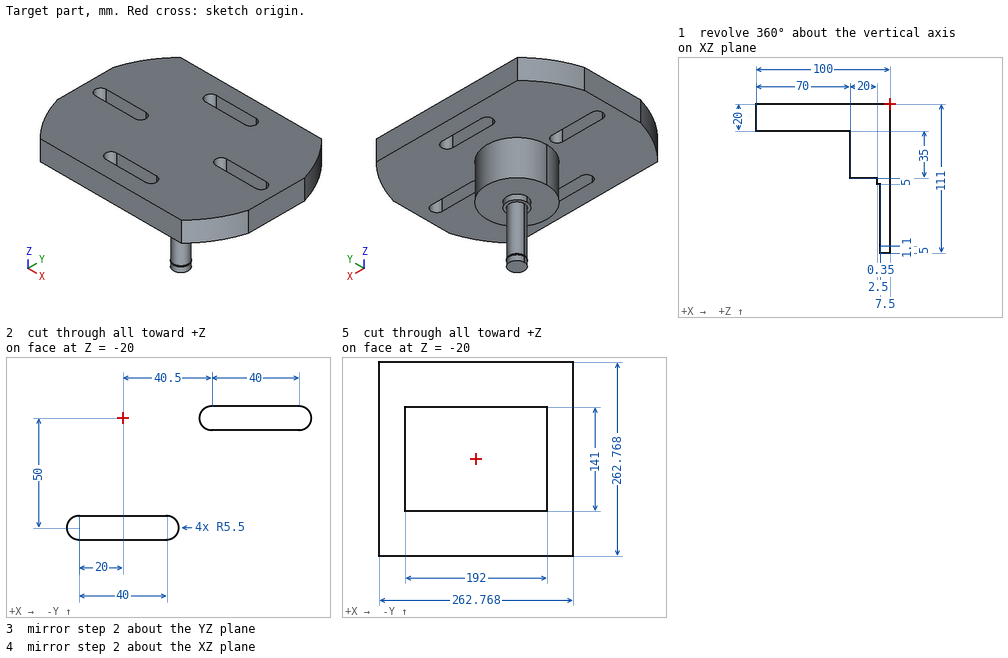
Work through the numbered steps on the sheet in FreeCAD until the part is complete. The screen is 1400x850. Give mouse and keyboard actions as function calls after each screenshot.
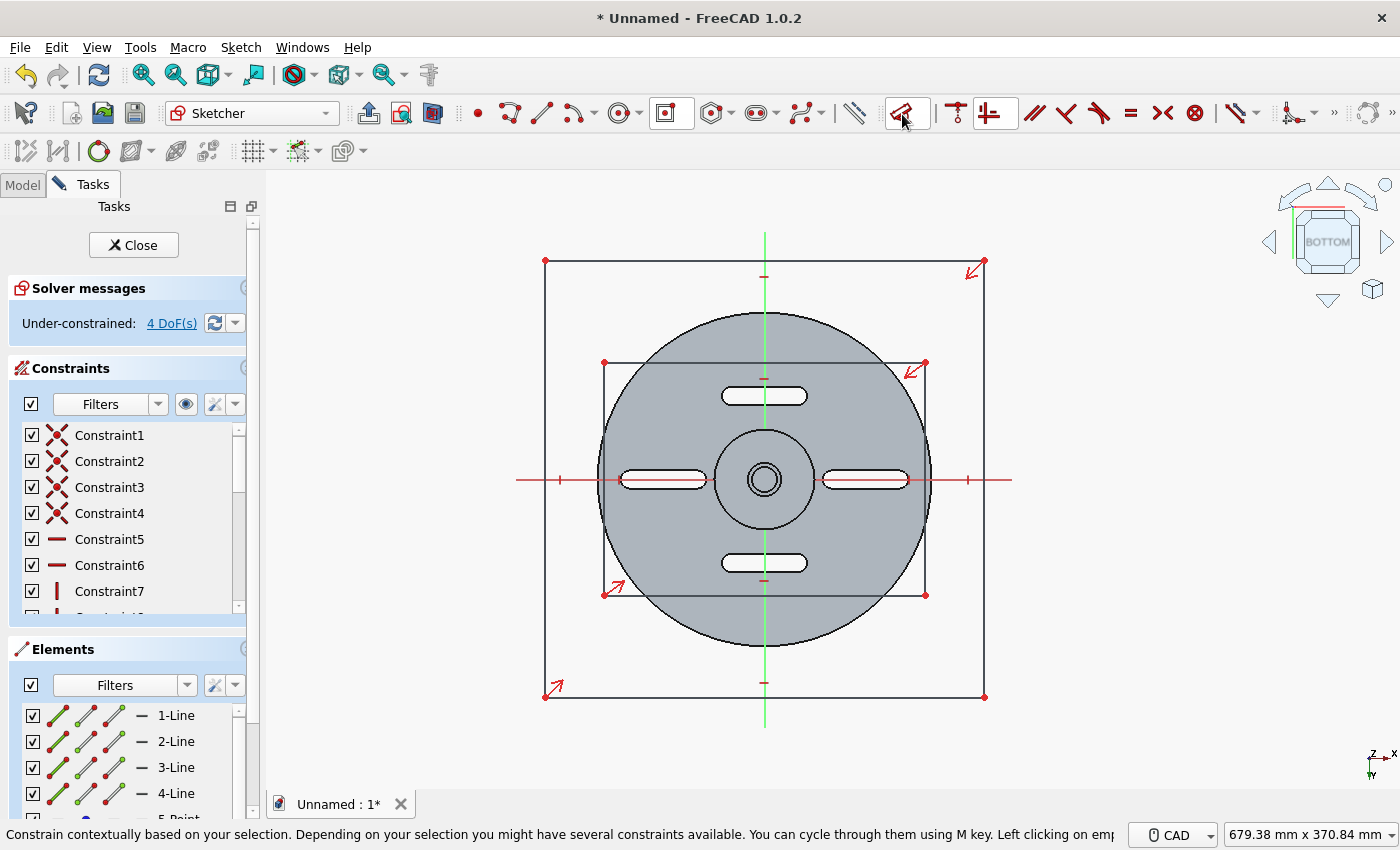
click(700, 596)
click(691, 630)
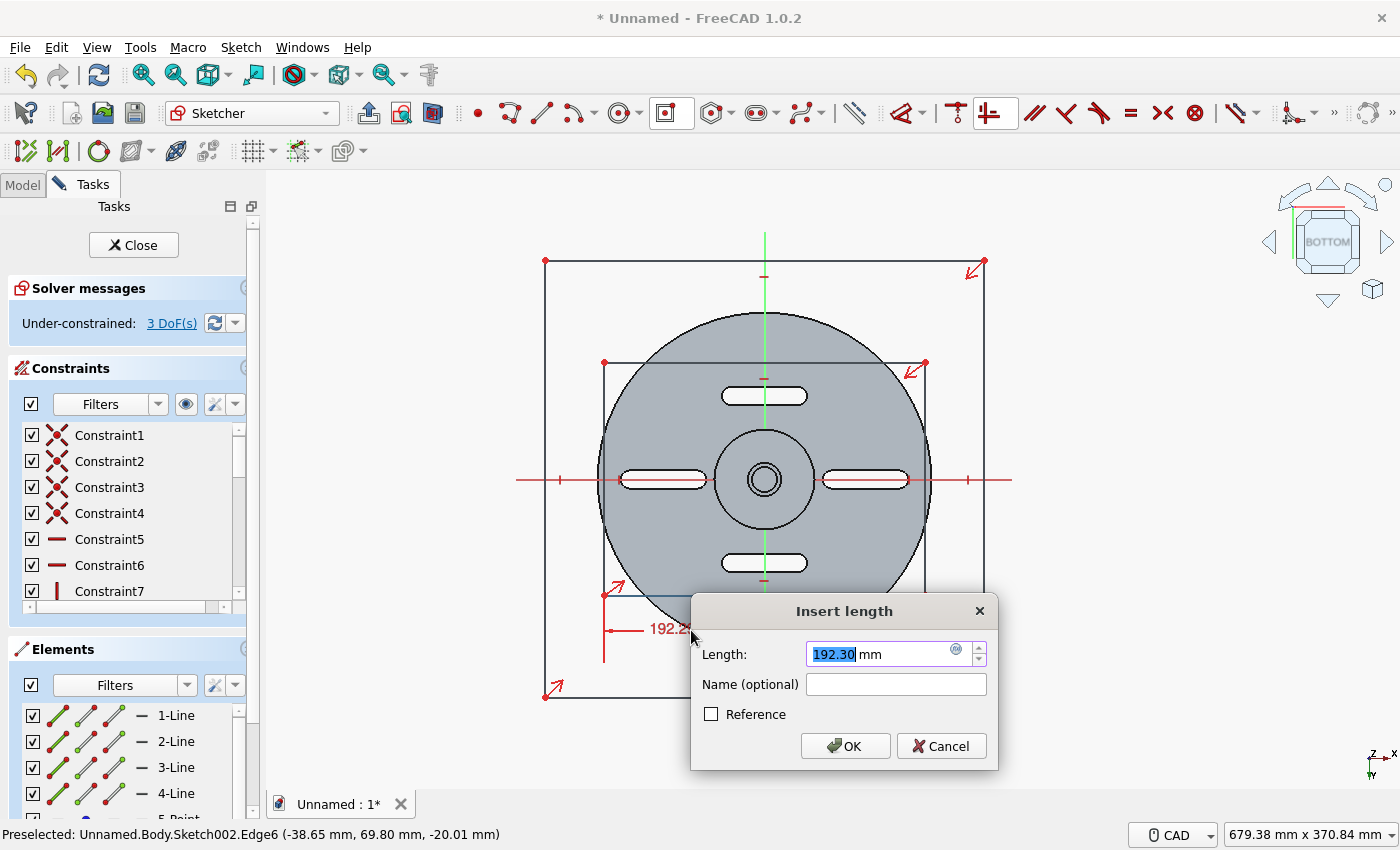
text(192)
key(Return)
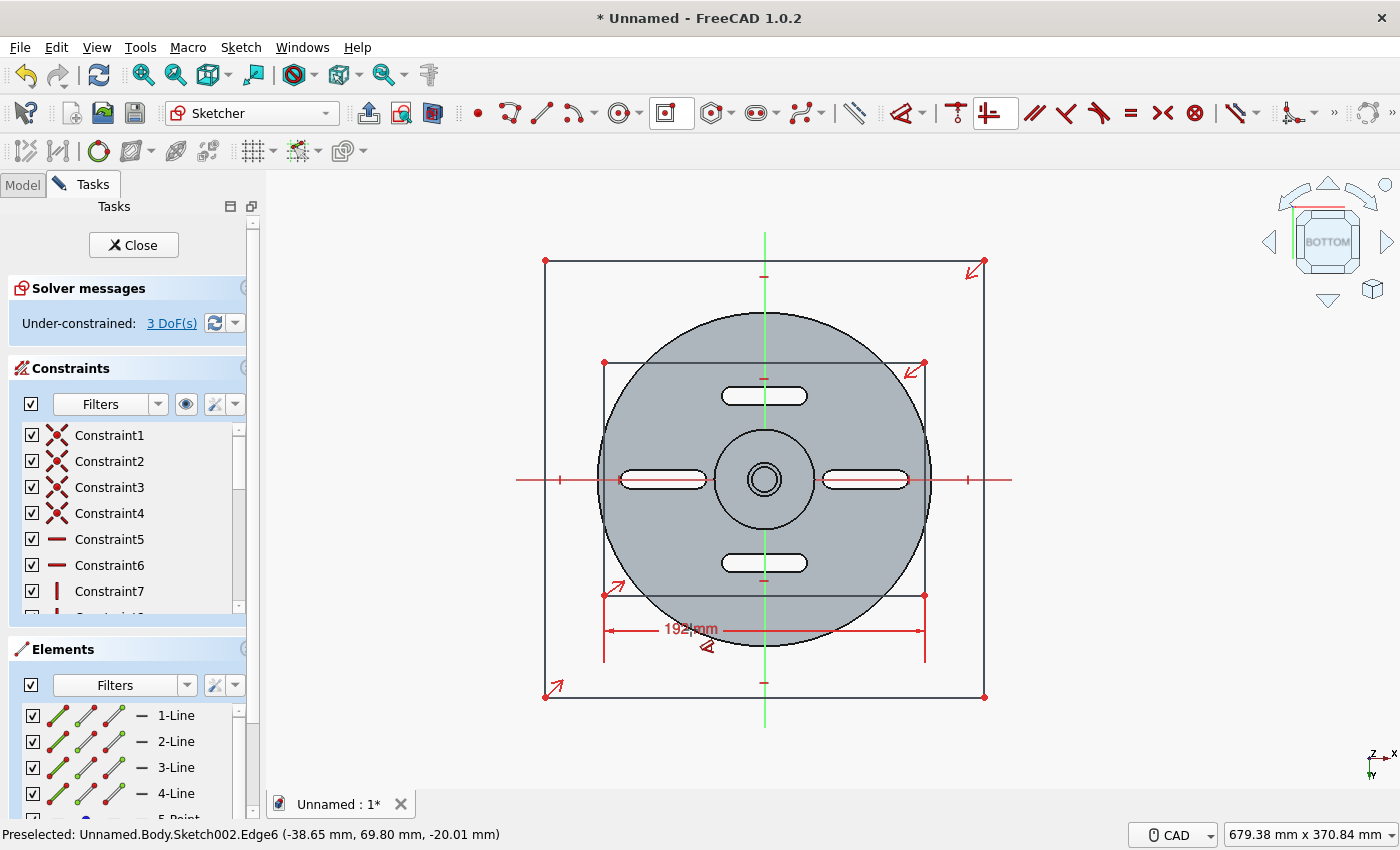
click(925, 526)
click(959, 426)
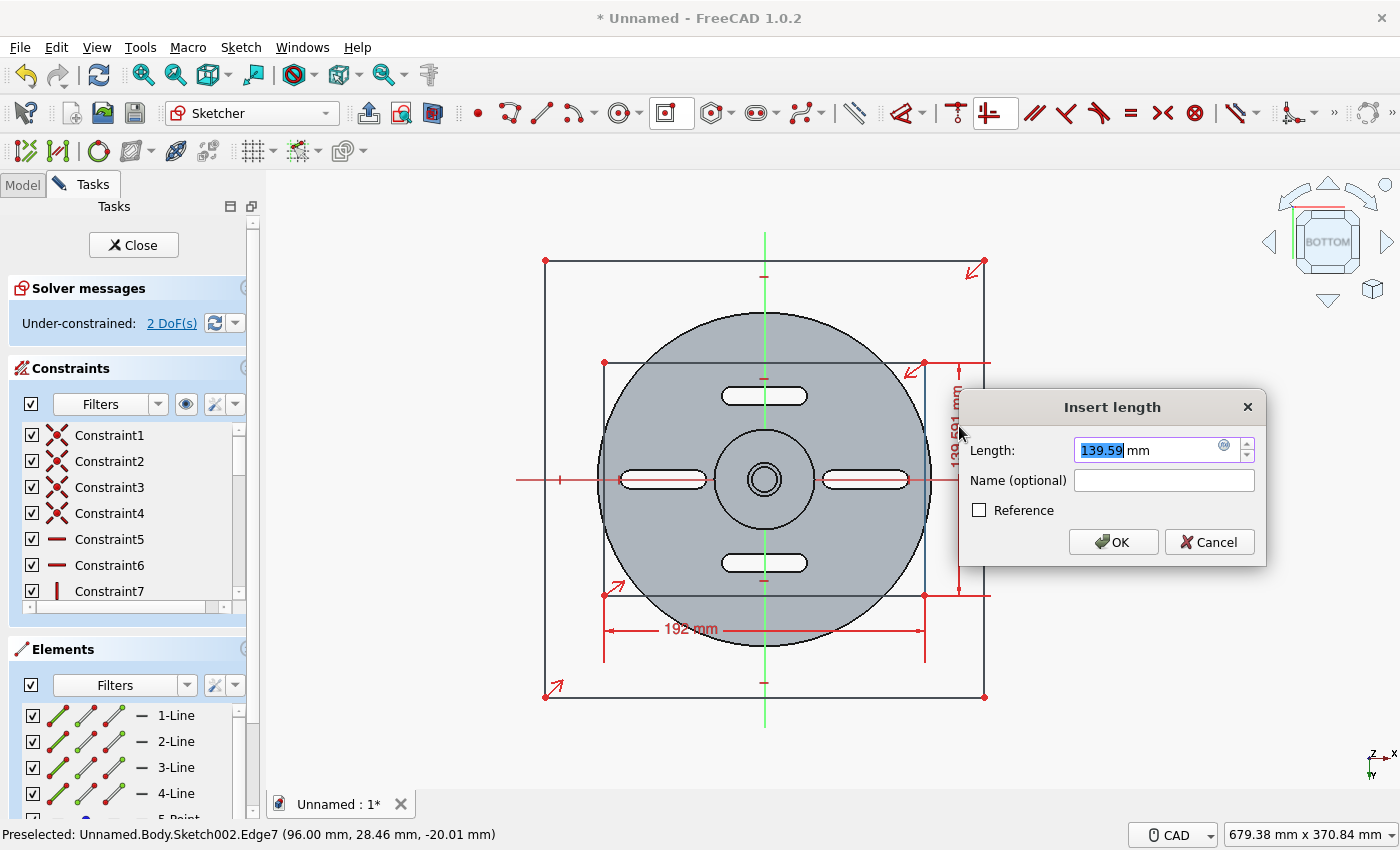
text(141)
key(Return)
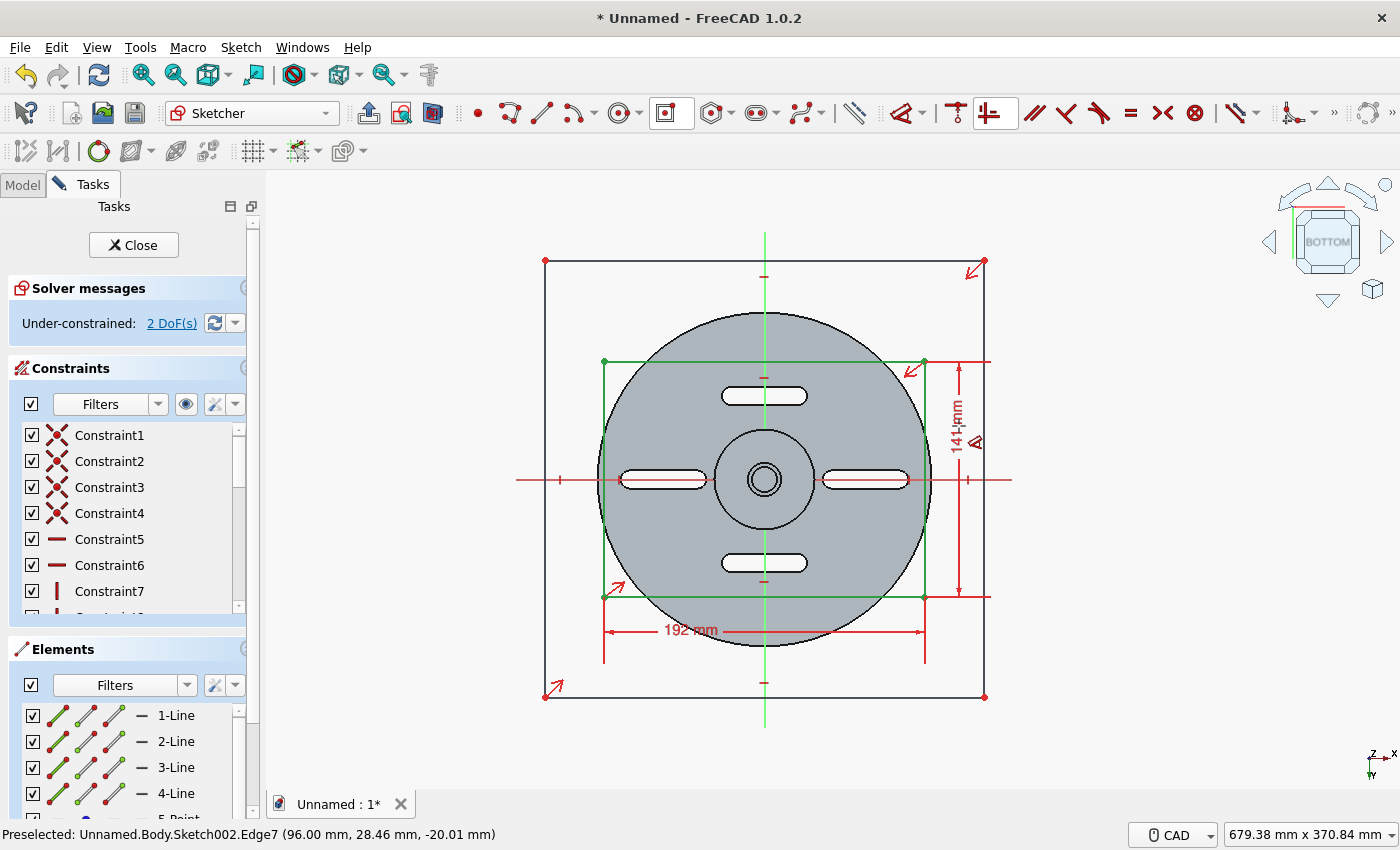
click(677, 698)
click(664, 732)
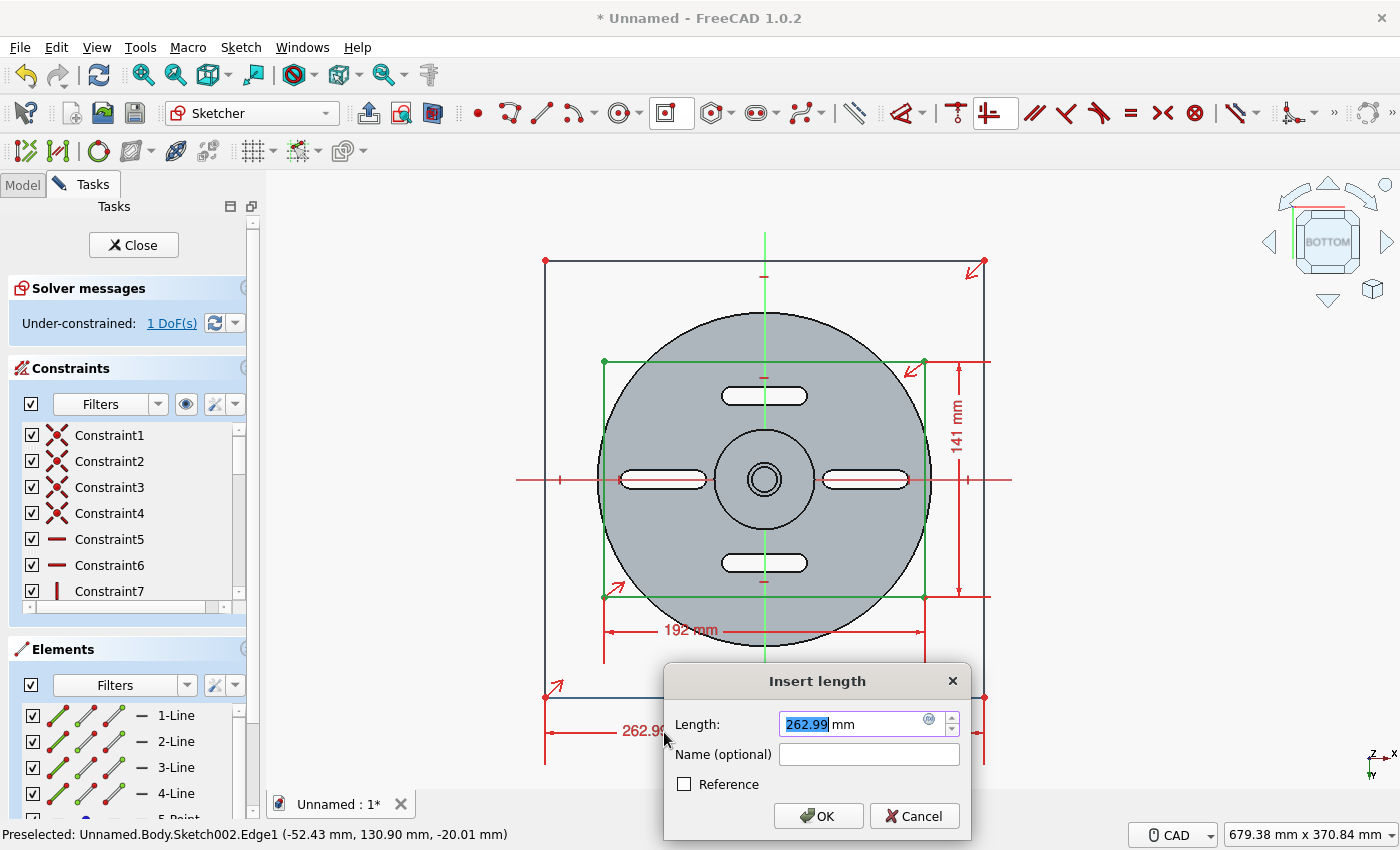
text(262.768)
key(Return)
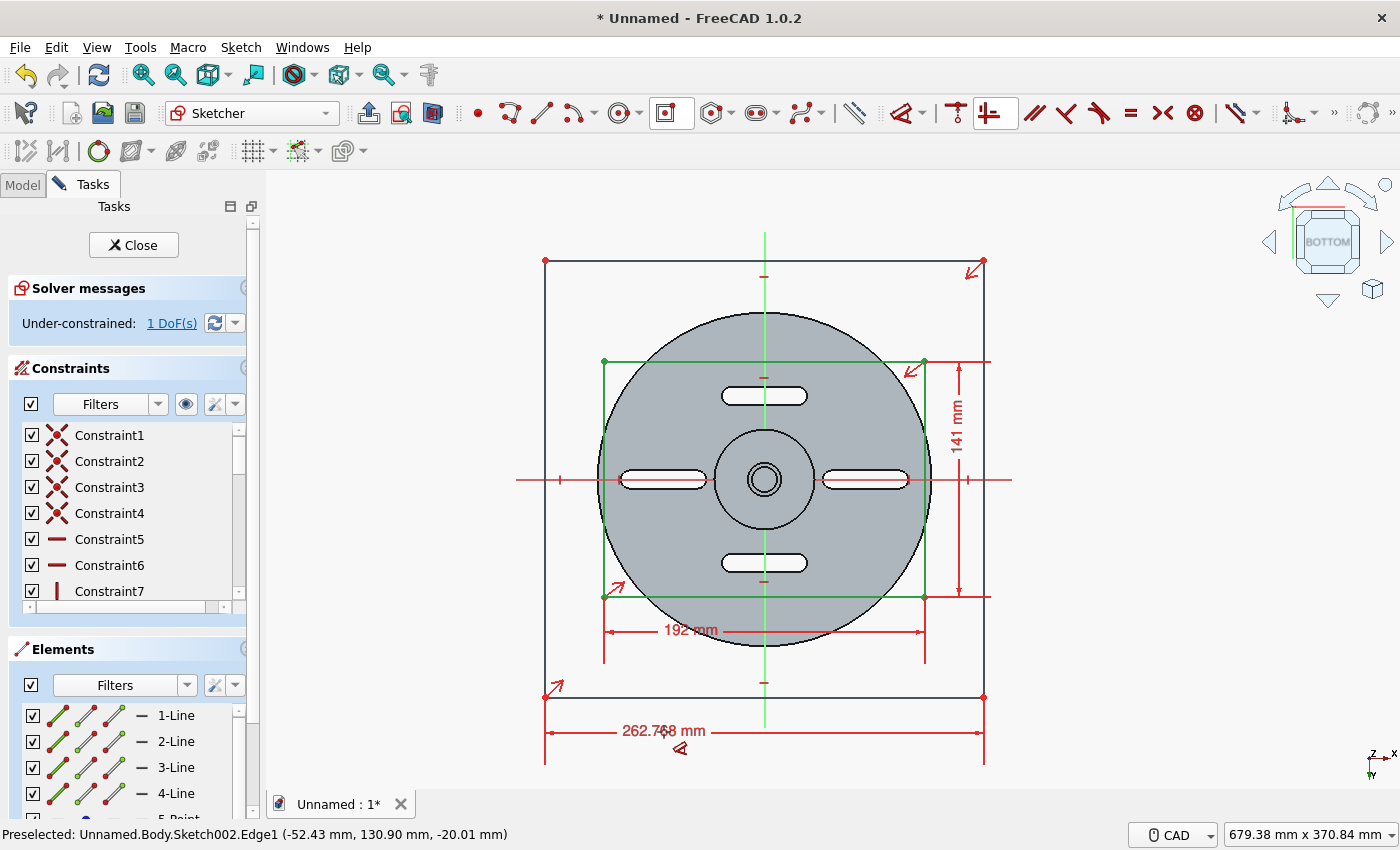
click(984, 567)
click(1018, 379)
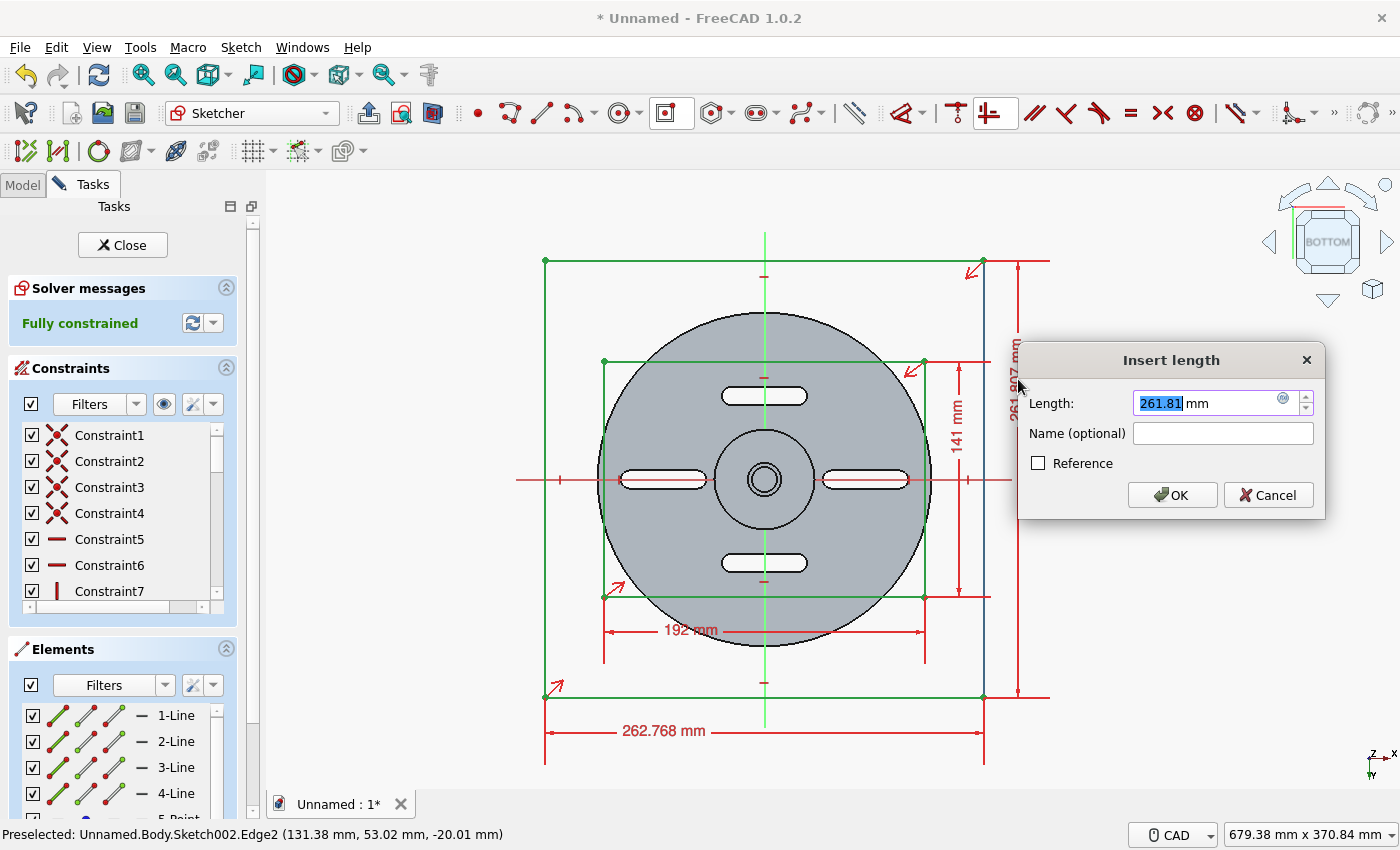
text(262.768)
key(Return)
key(Escape)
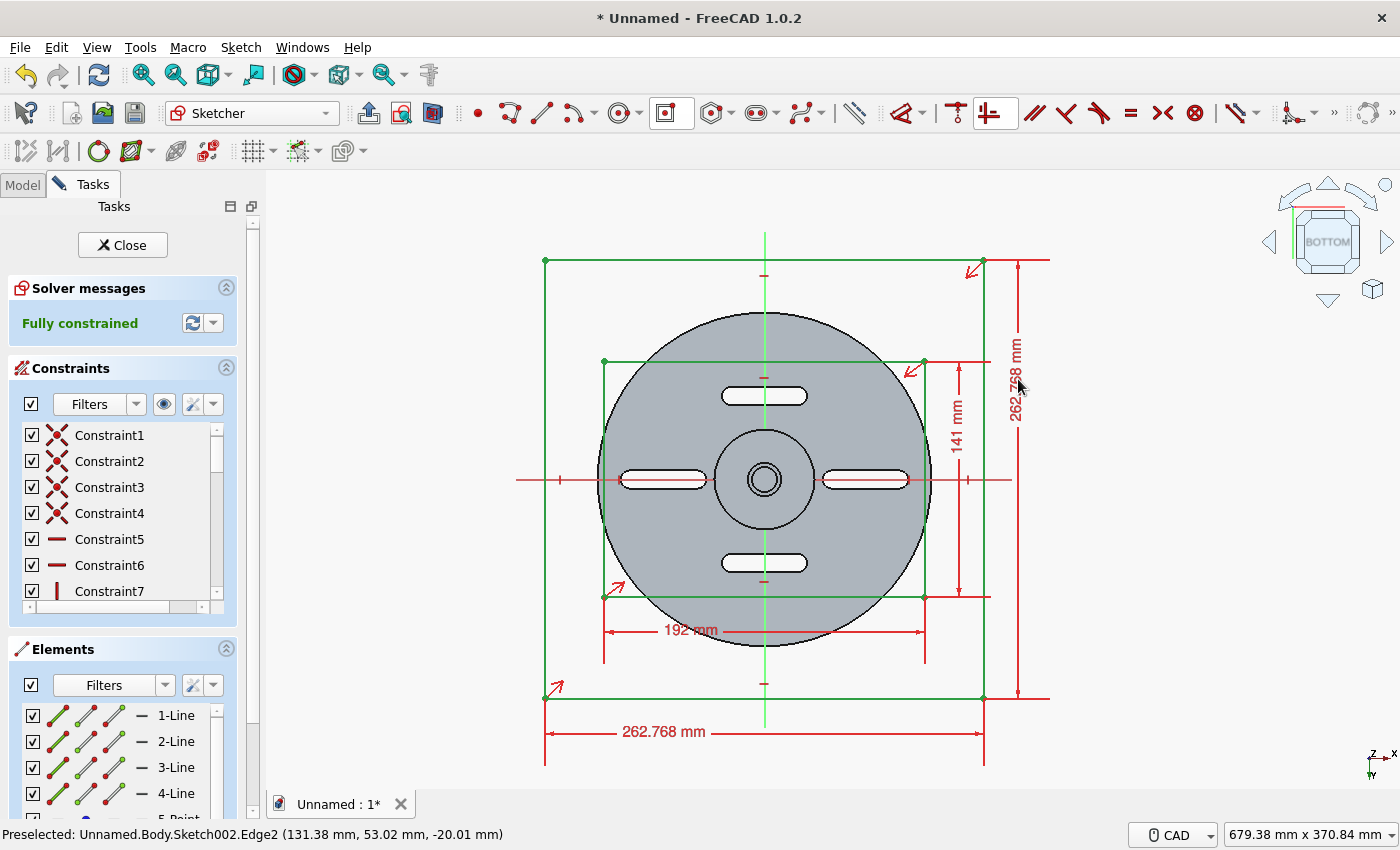
click(123, 245)